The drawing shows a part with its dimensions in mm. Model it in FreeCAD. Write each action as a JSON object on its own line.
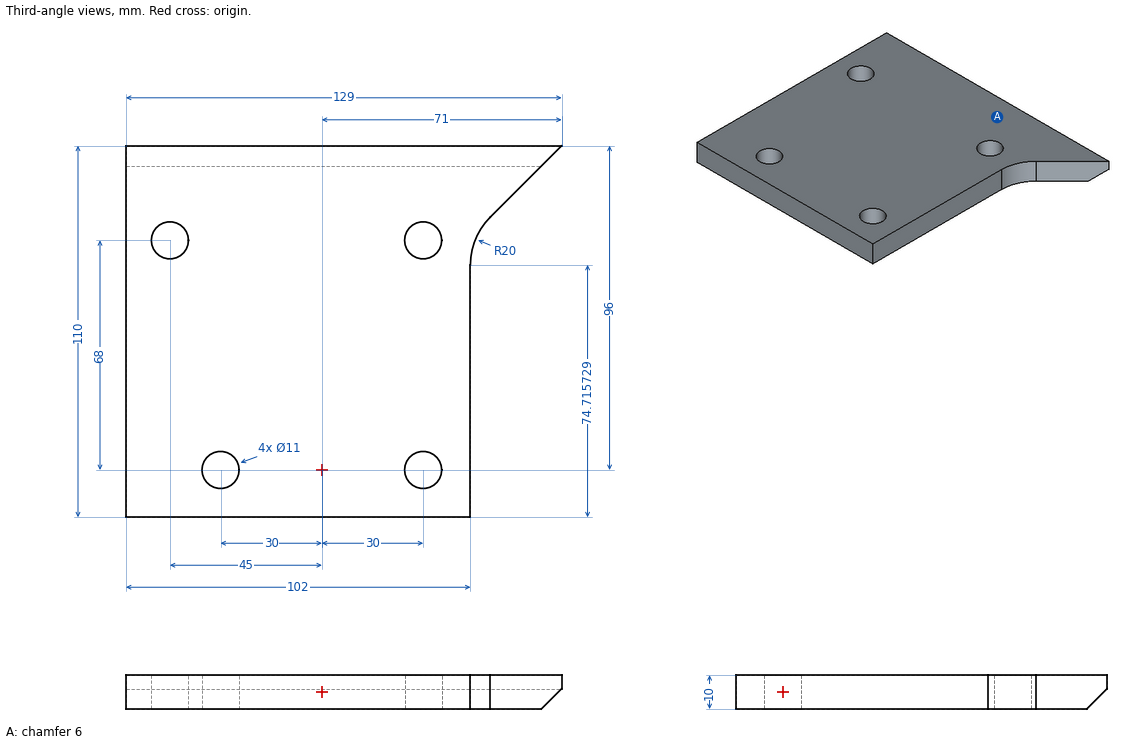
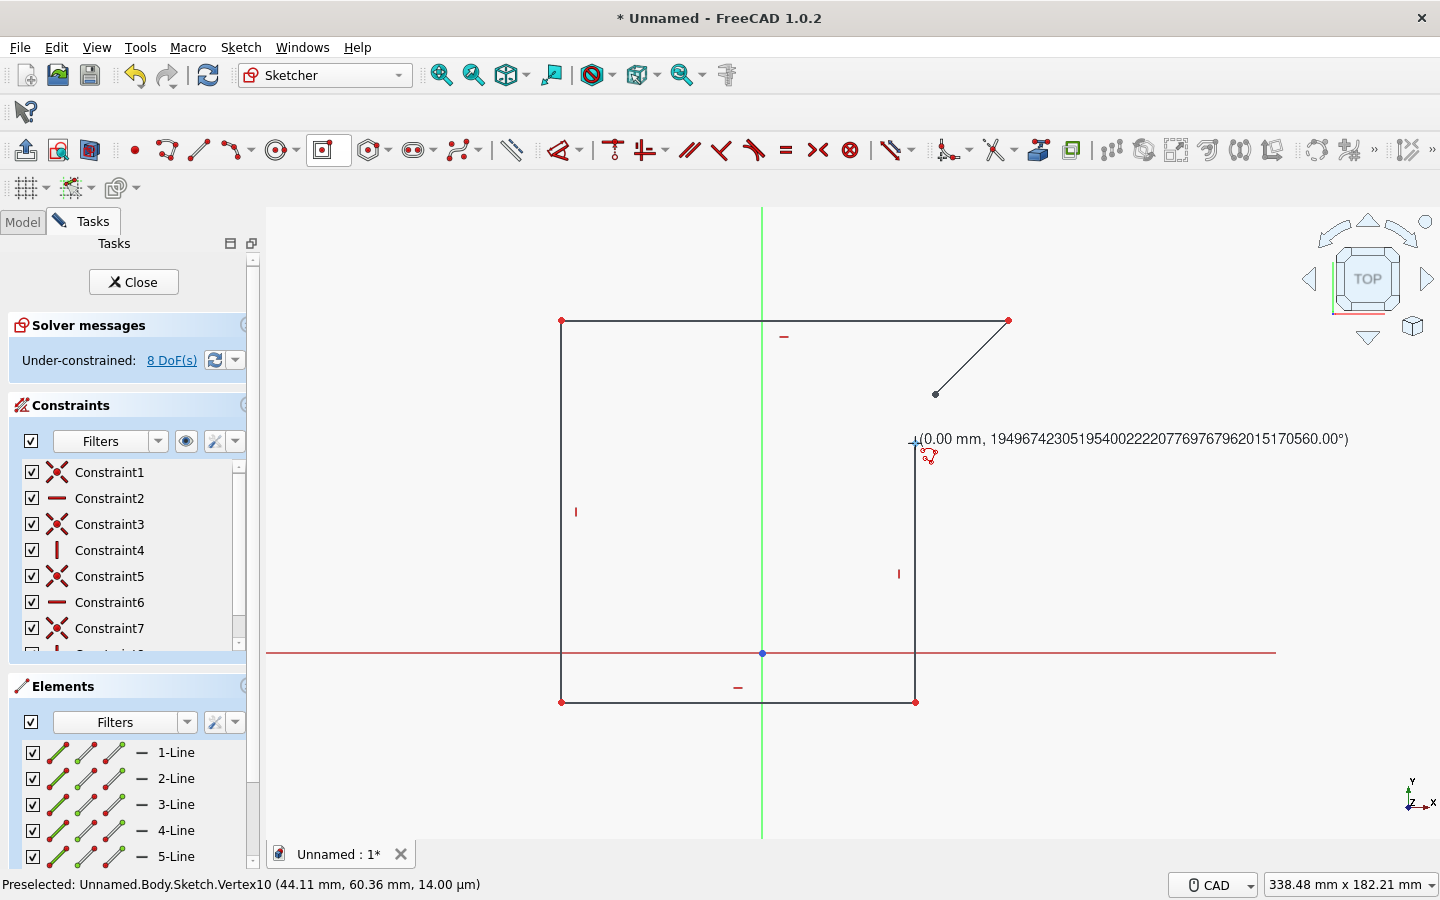
{"action": "left_click", "coordinate": [232, 150]}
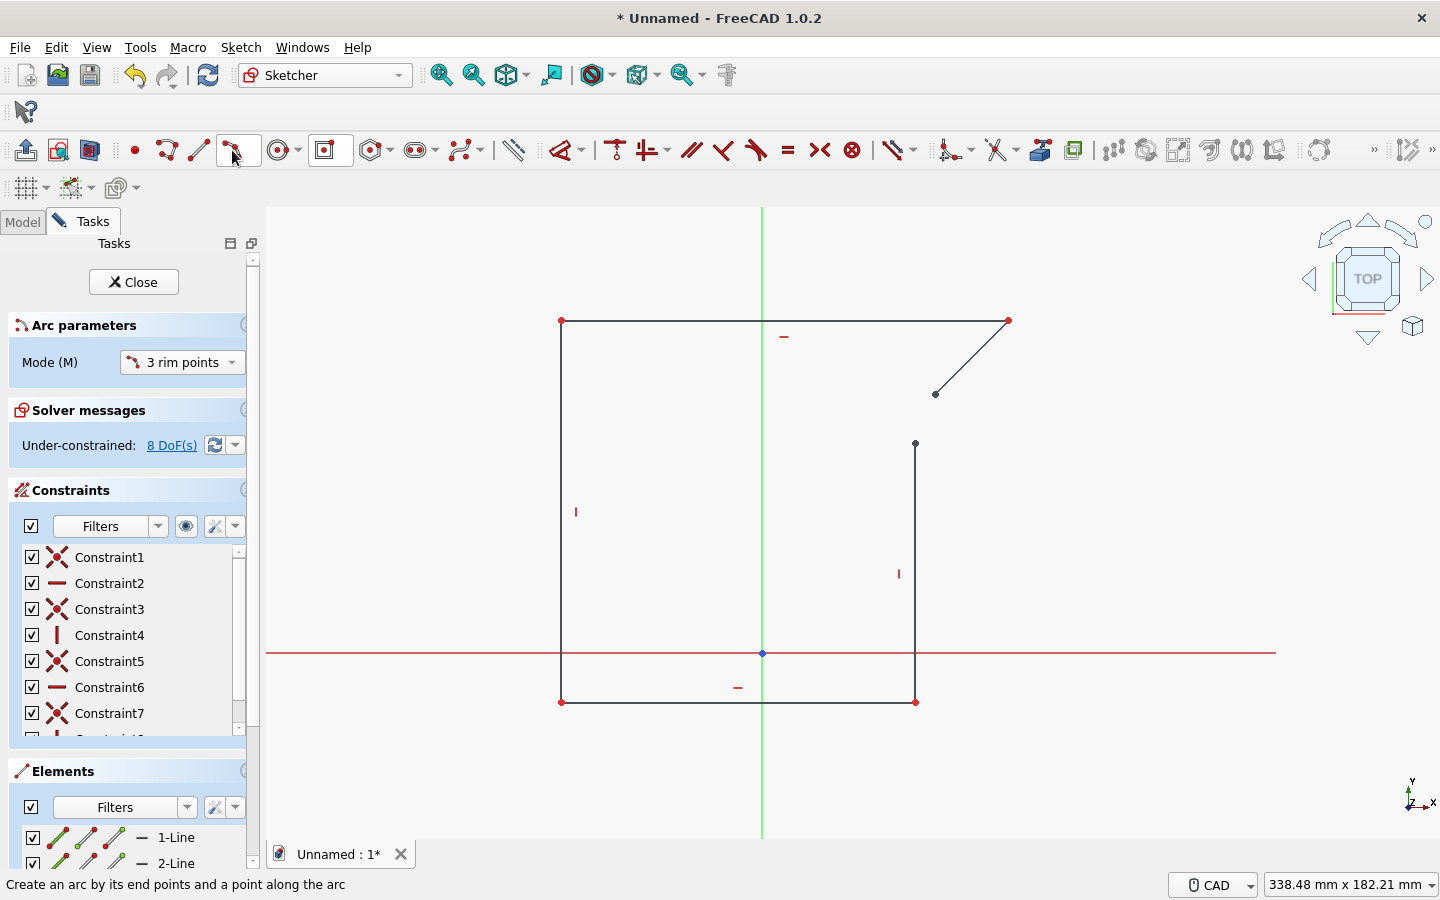
{"action": "left_click", "coordinate": [915, 444]}
{"action": "left_click", "coordinate": [935, 395]}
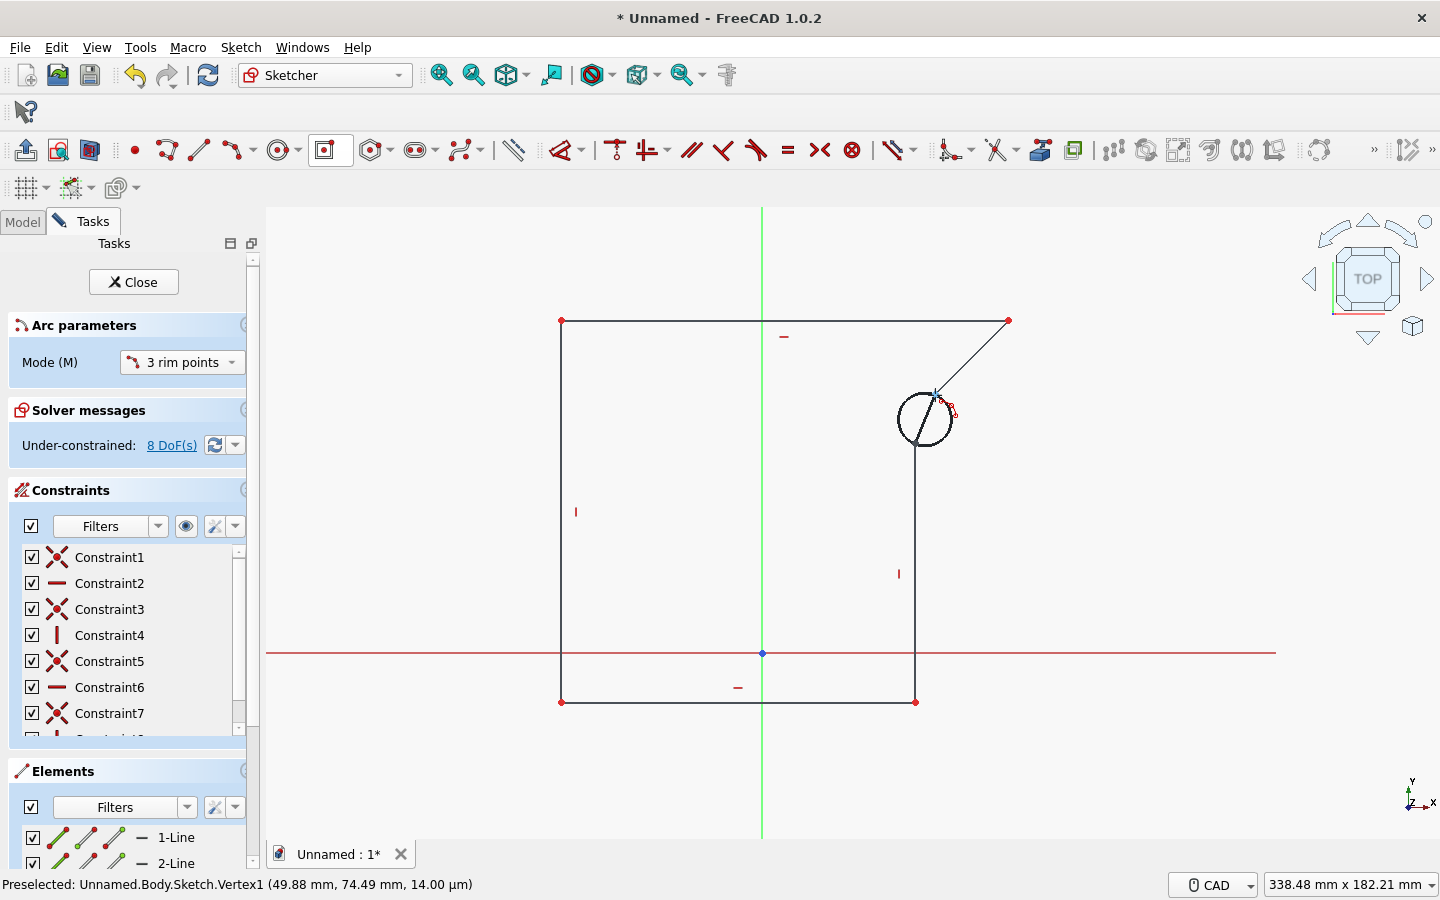
{"action": "scroll", "coordinate": [920, 416], "scroll_direction": "up", "scroll_amount": 6}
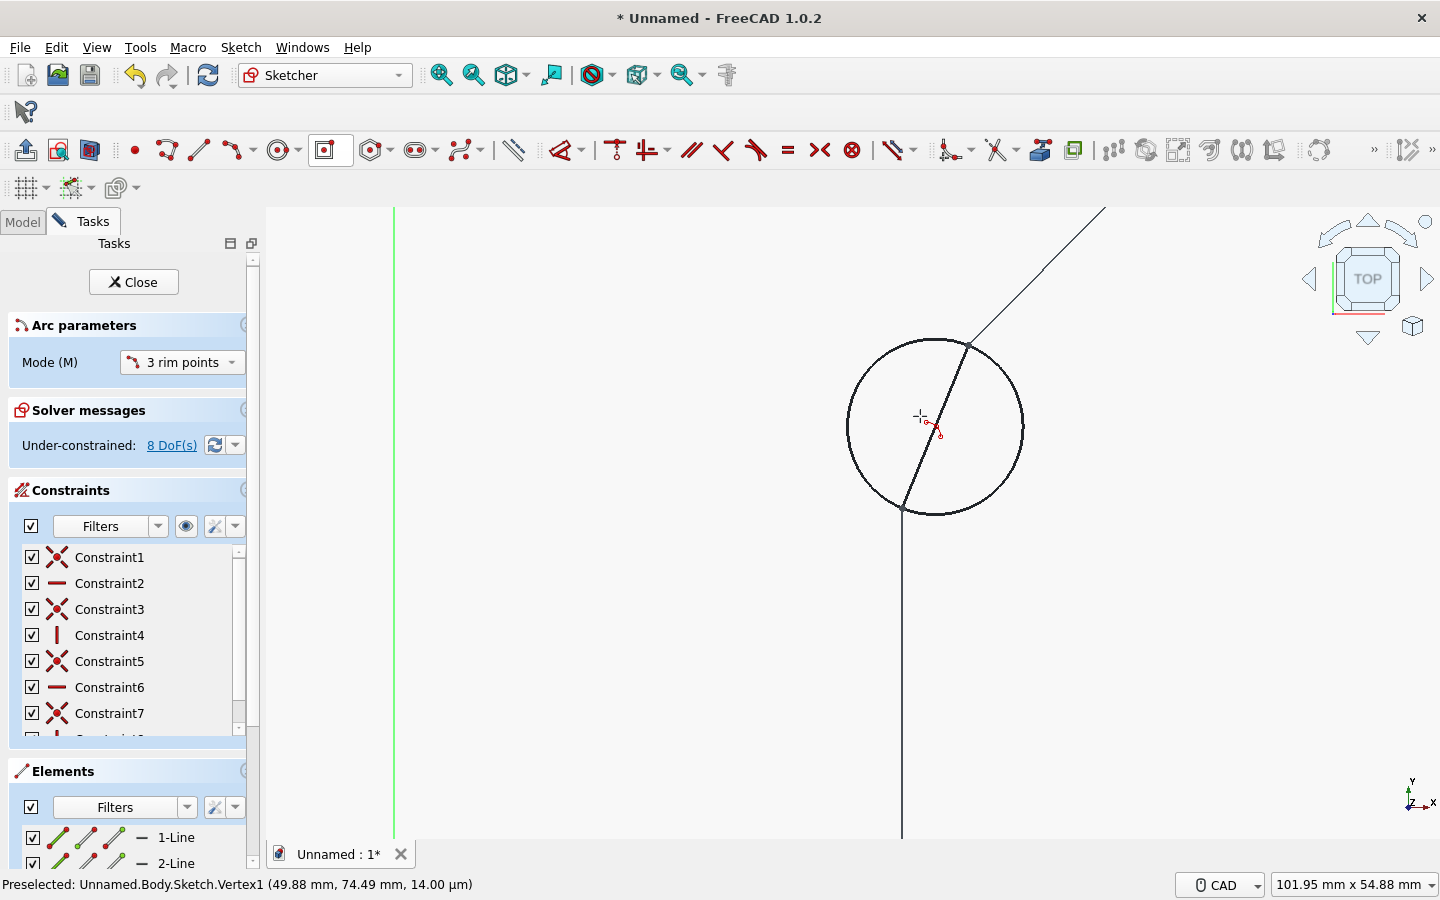
{"action": "left_click", "coordinate": [918, 416]}
{"action": "key", "text": "Escape"}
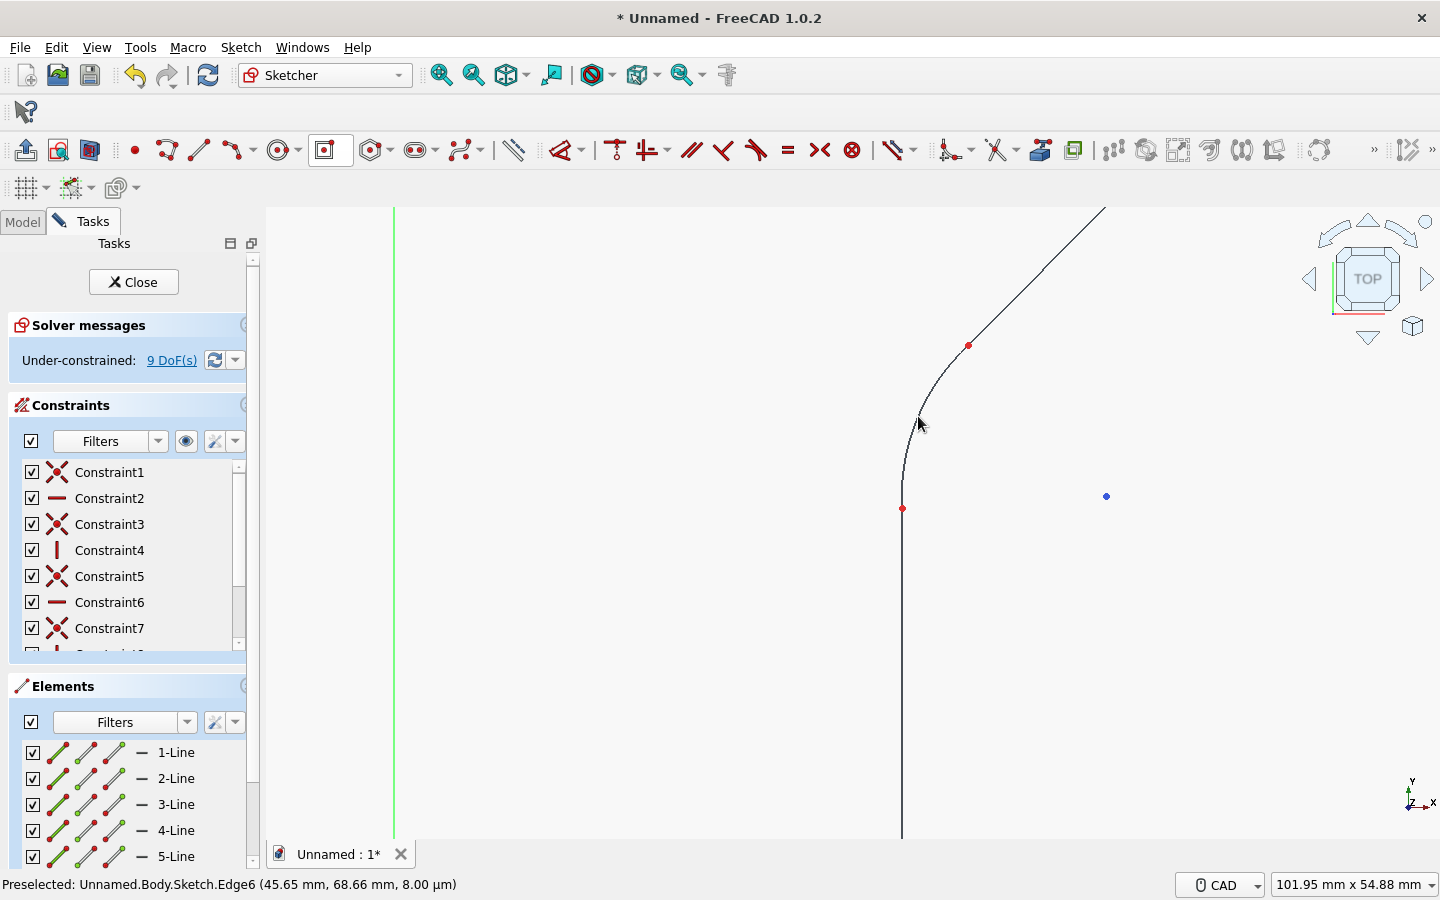
{"action": "left_click", "coordinate": [1041, 272]}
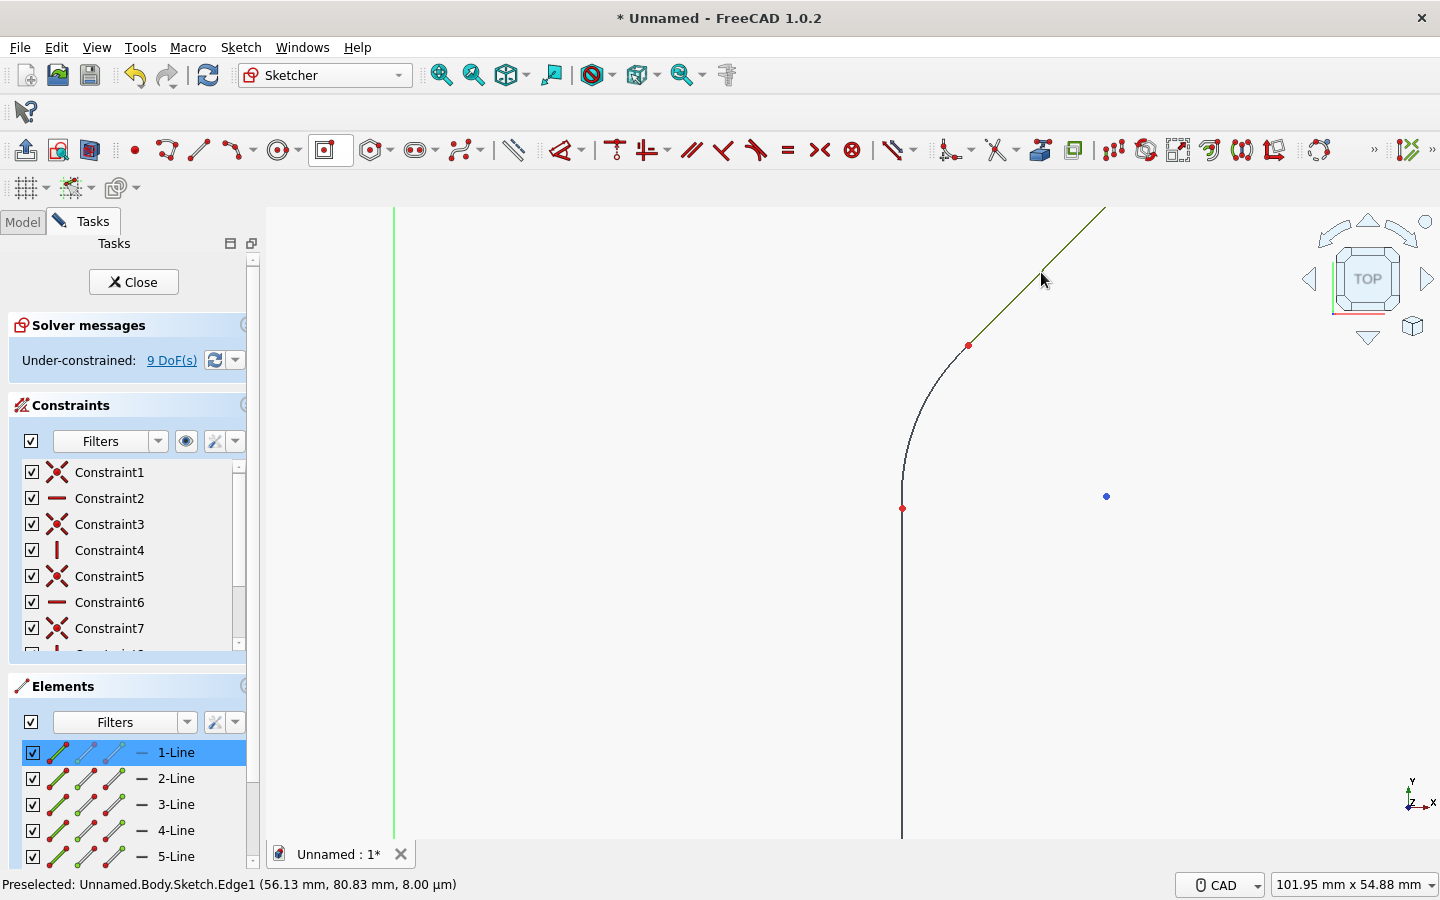
{"action": "left_click", "coordinate": [934, 387]}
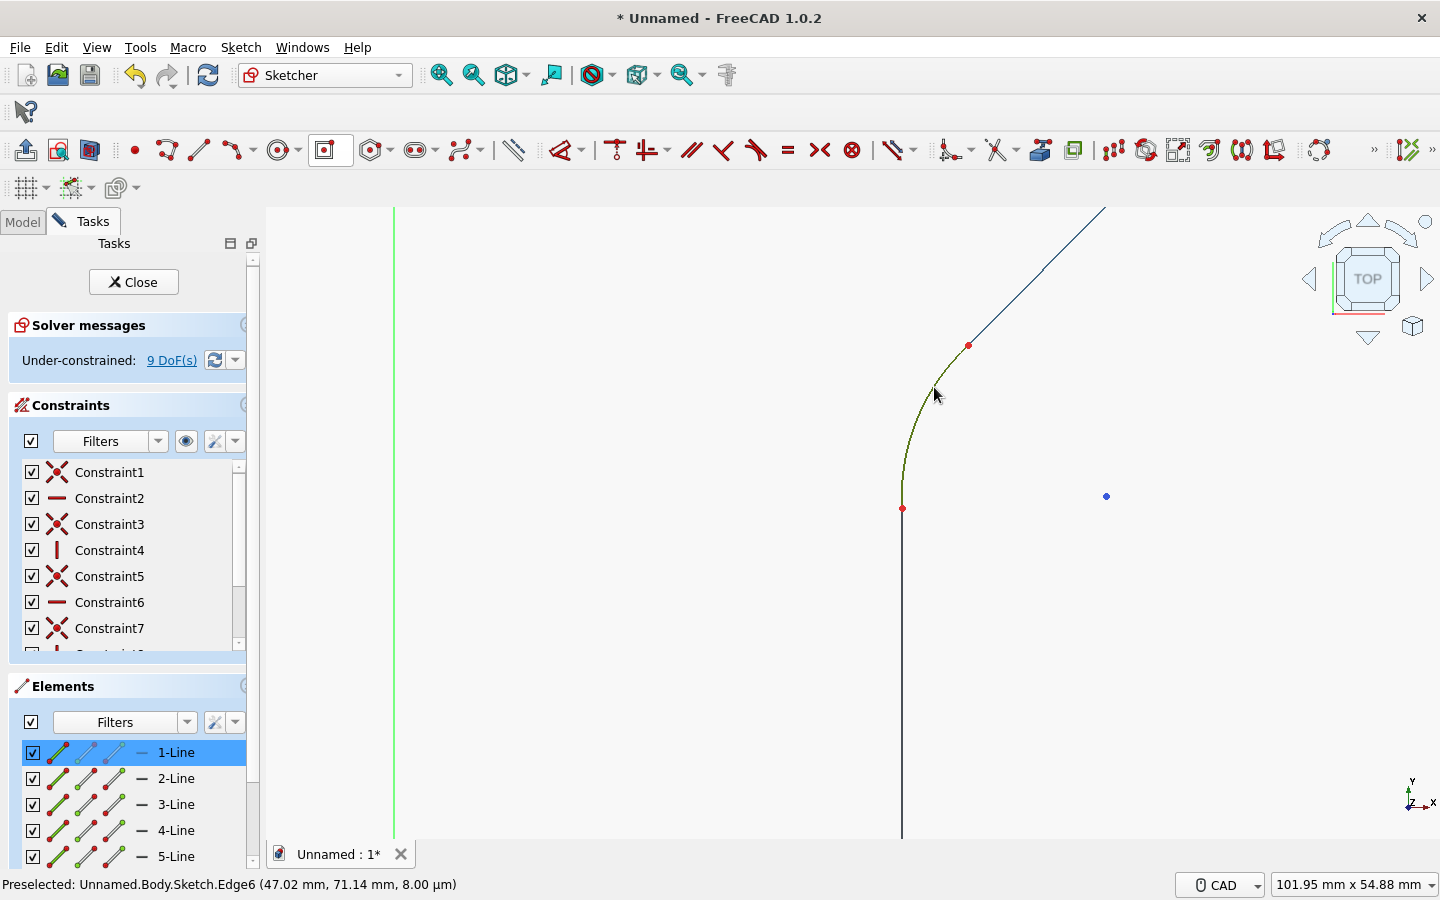
{"action": "key", "text": "t"}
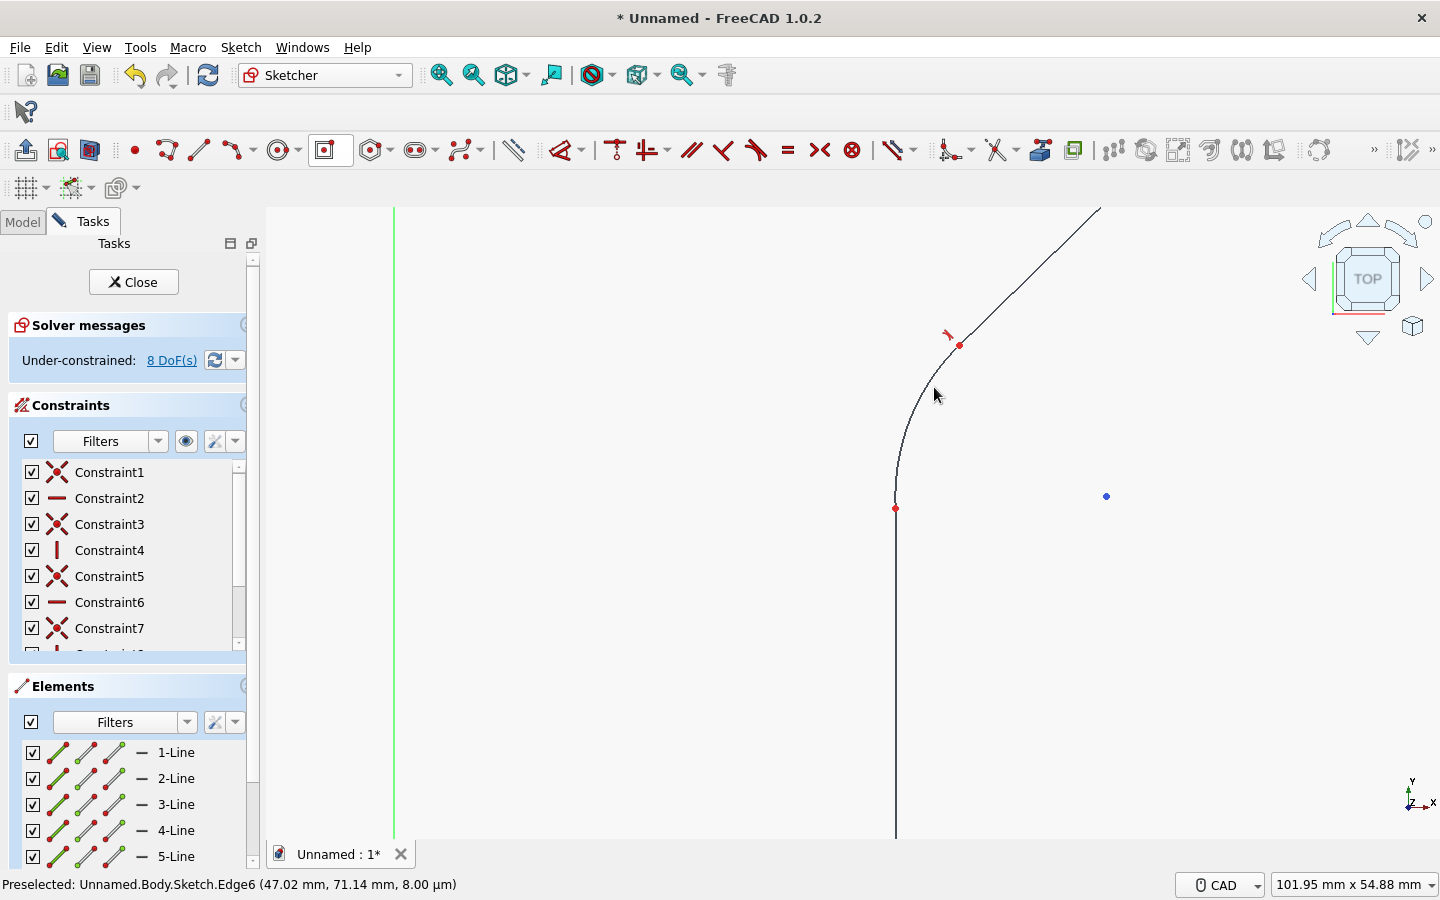
{"action": "left_click", "coordinate": [896, 766]}